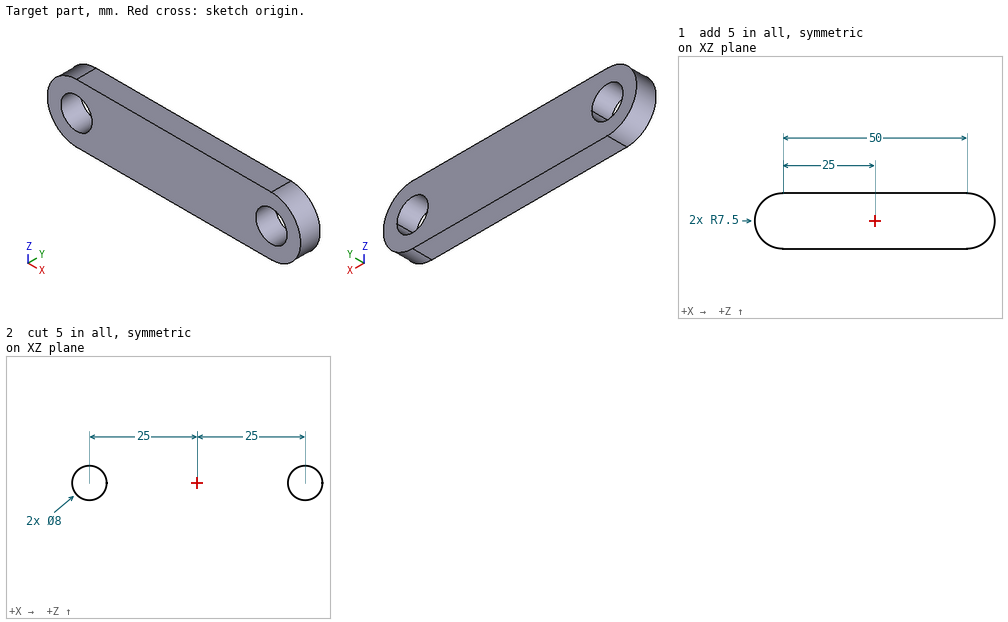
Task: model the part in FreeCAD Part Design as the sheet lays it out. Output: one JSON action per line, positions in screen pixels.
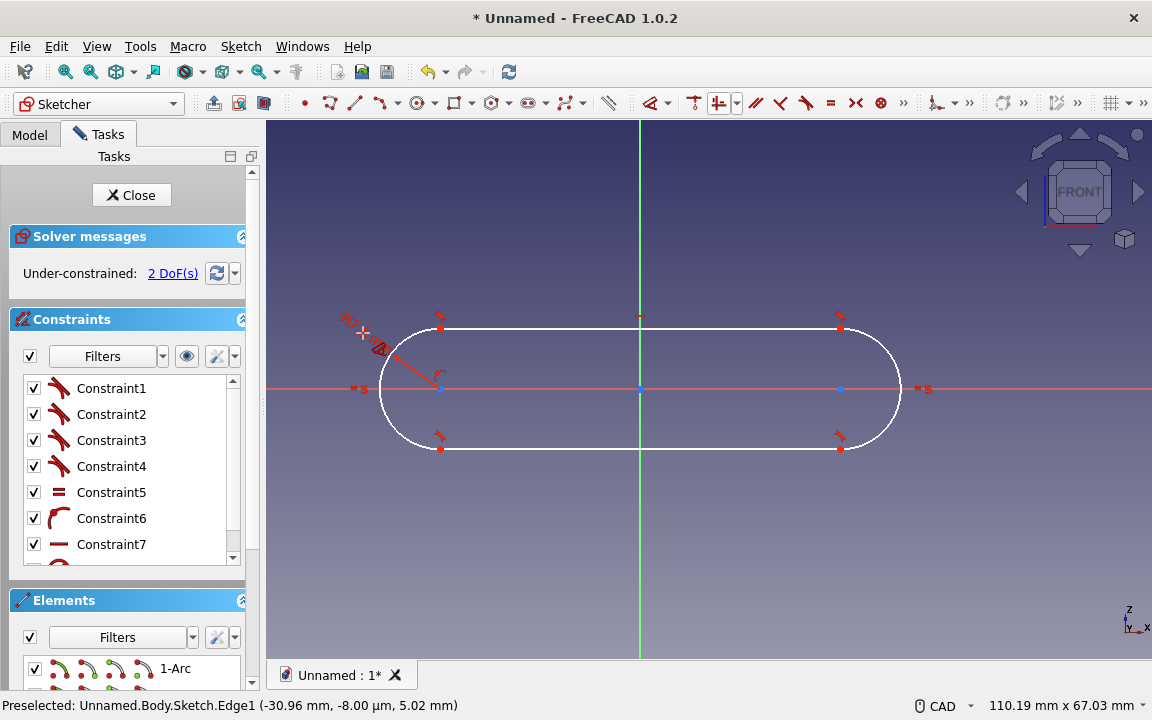
{"action": "left_click", "coordinate": [560, 329]}
{"action": "left_click", "coordinate": [548, 295]}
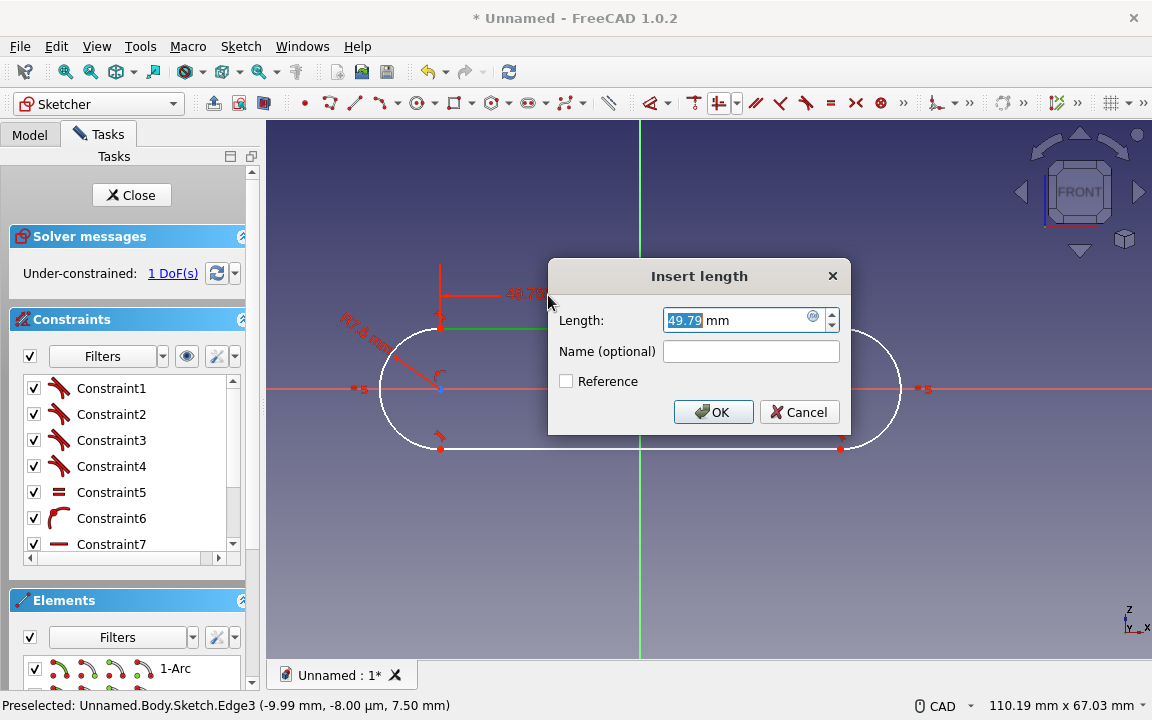
{"action": "type", "text": "50"}
{"action": "key", "text": "Return"}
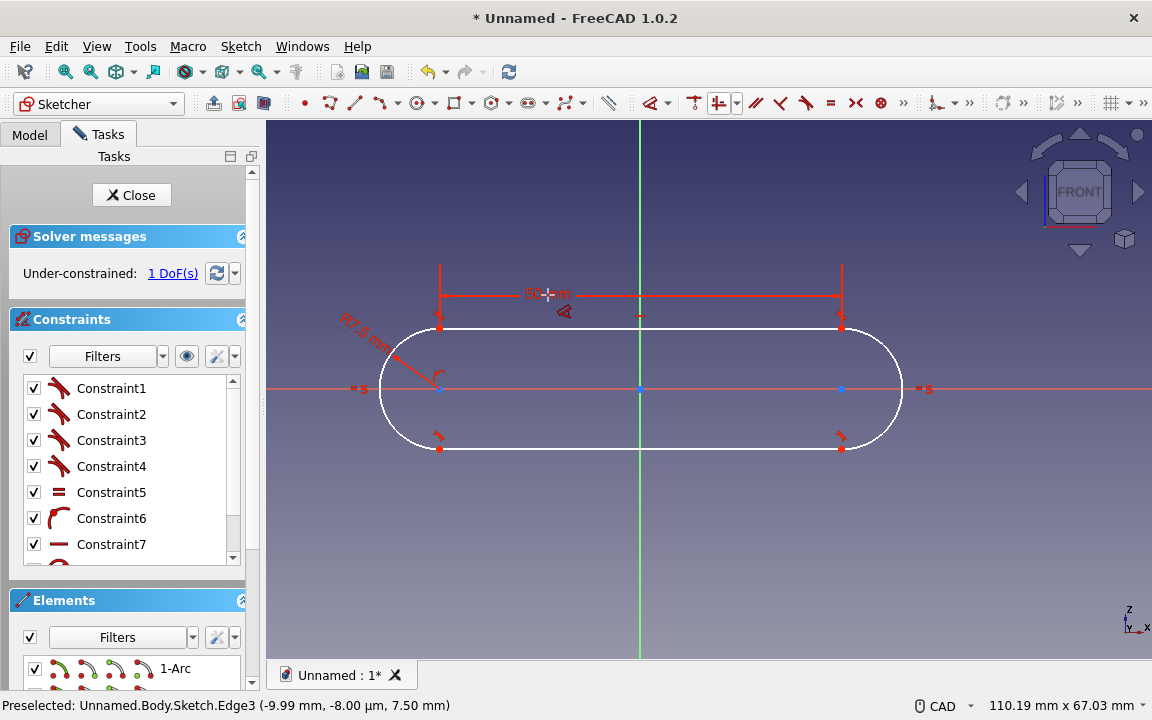
{"action": "left_click", "coordinate": [440, 329]}
{"action": "left_click", "coordinate": [470, 295]}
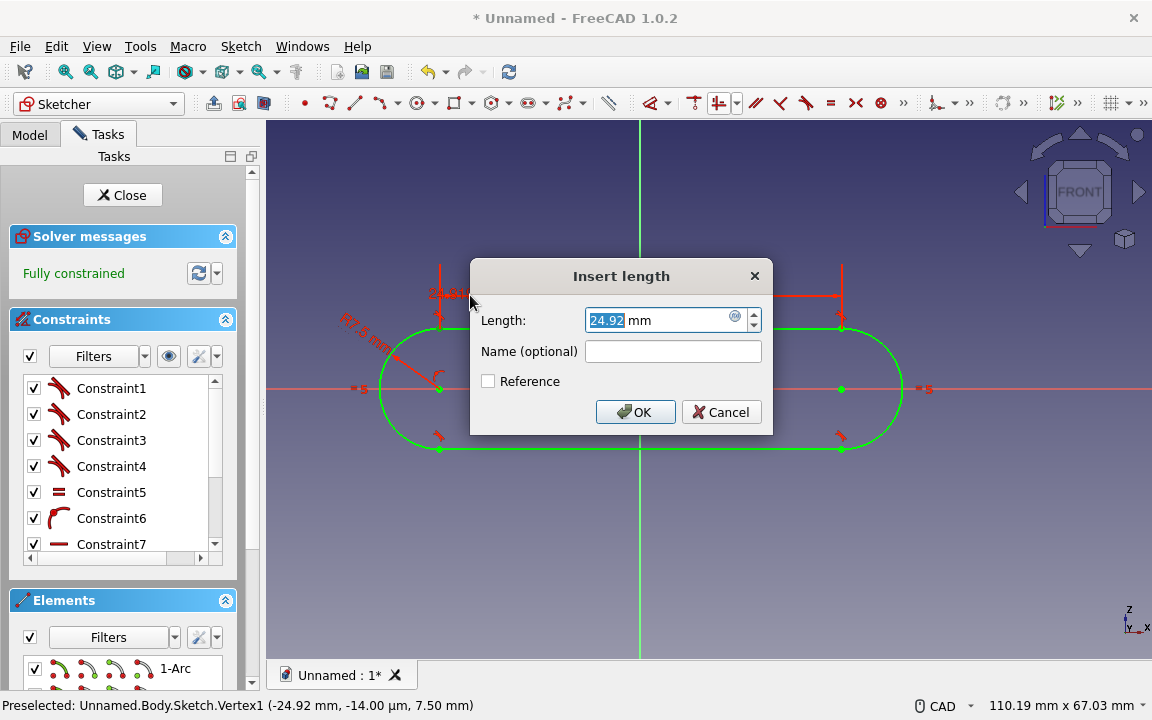
{"action": "type", "text": "25"}
{"action": "key", "text": "Return"}
{"action": "key", "text": "Escape"}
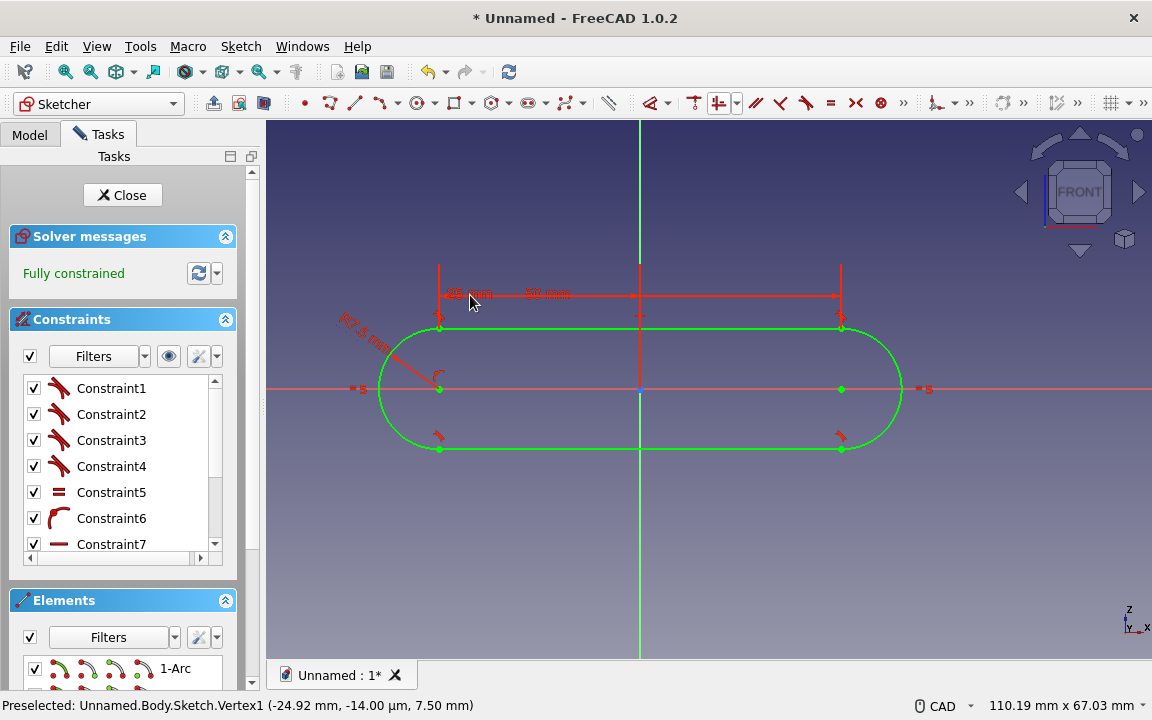
{"action": "left_click", "coordinate": [123, 195]}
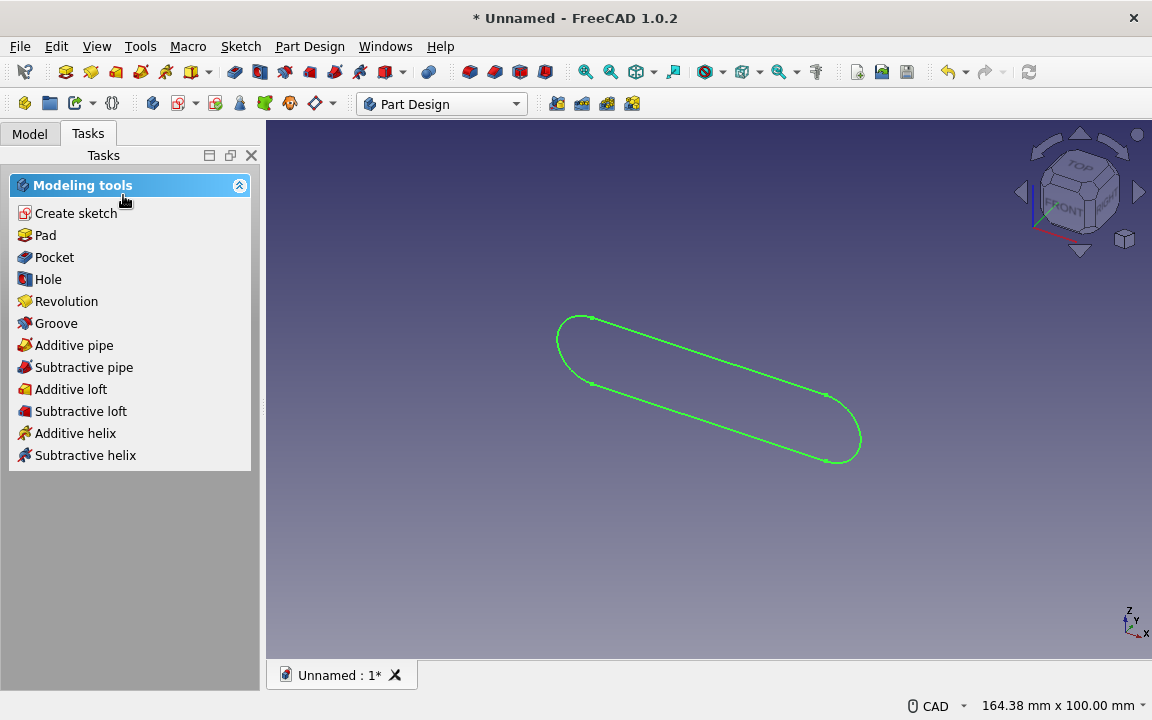
{"action": "left_click", "coordinate": [66, 72]}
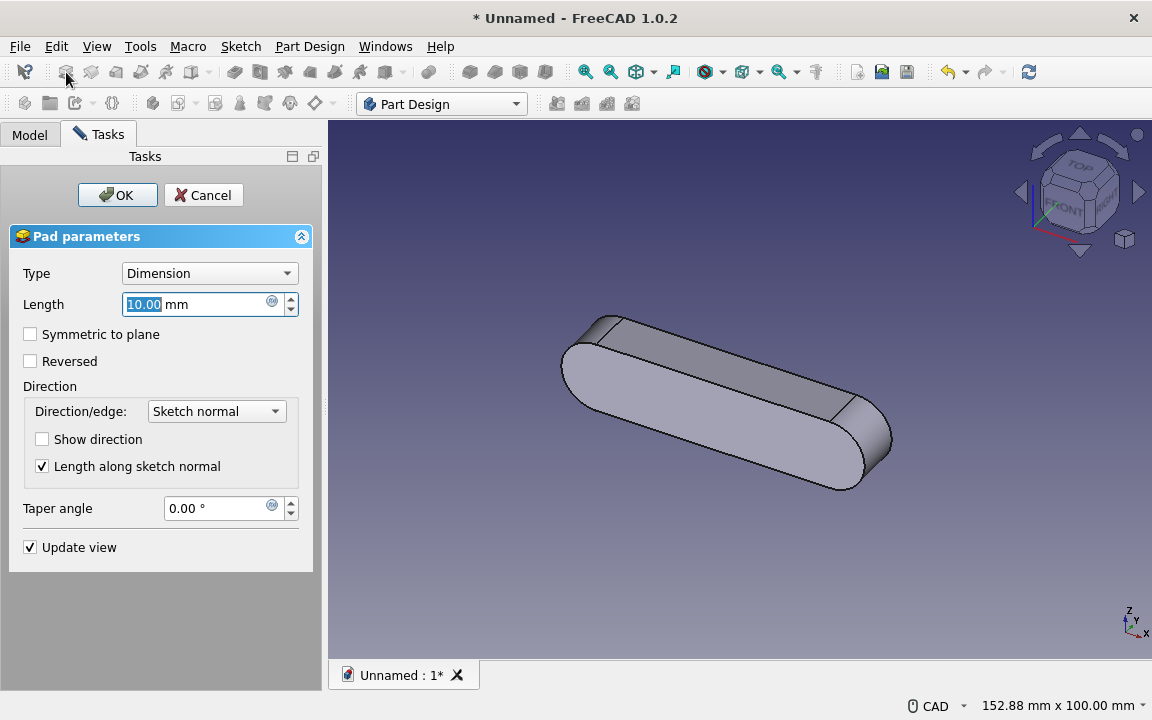
{"action": "type", "text": "5"}
{"action": "key", "text": "Tab"}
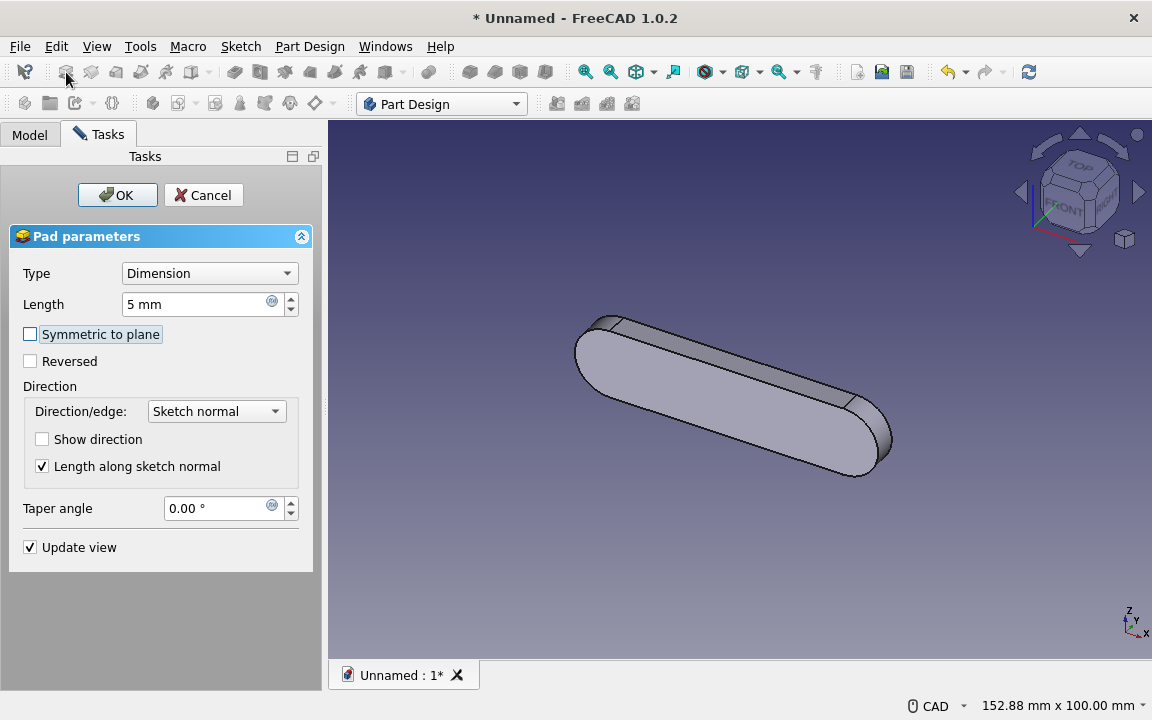
{"action": "left_click", "coordinate": [31, 334]}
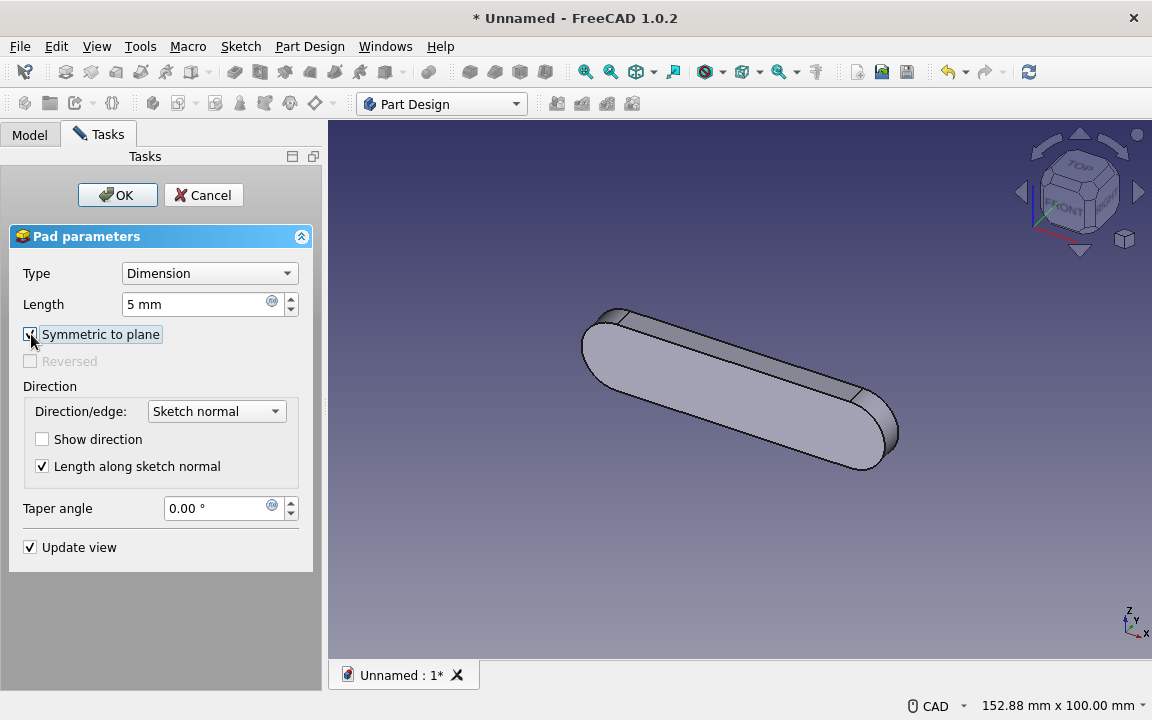
{"action": "left_click", "coordinate": [118, 195]}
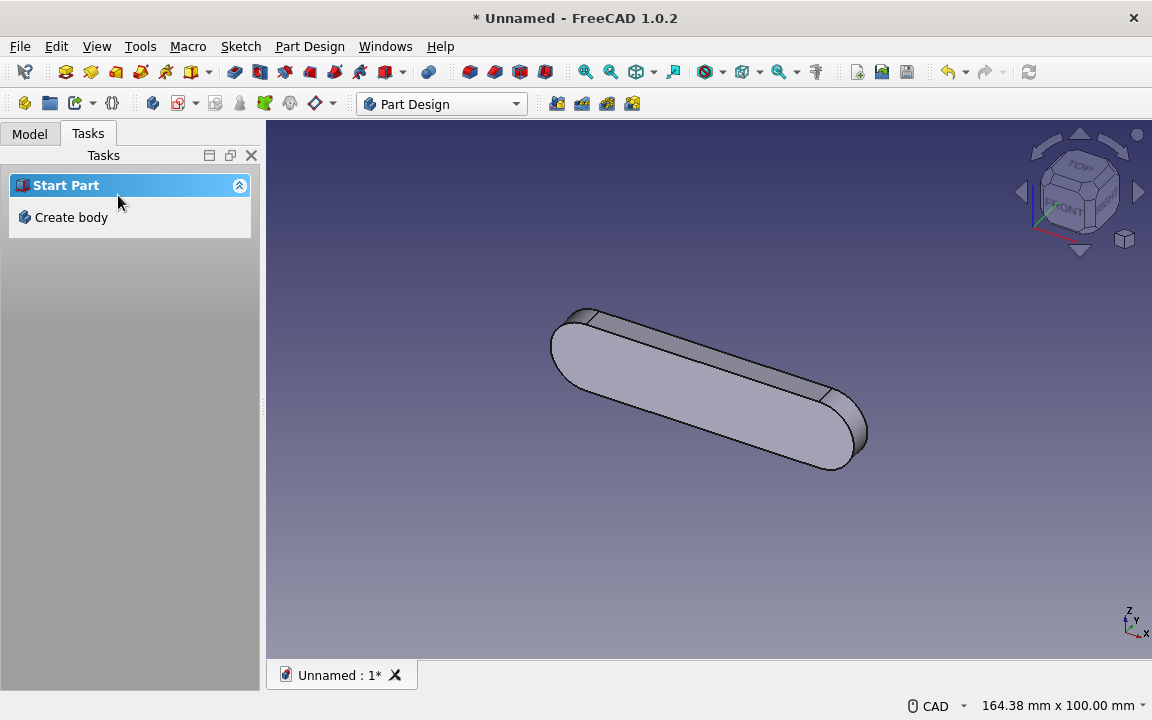
{"action": "left_click", "coordinate": [586, 72]}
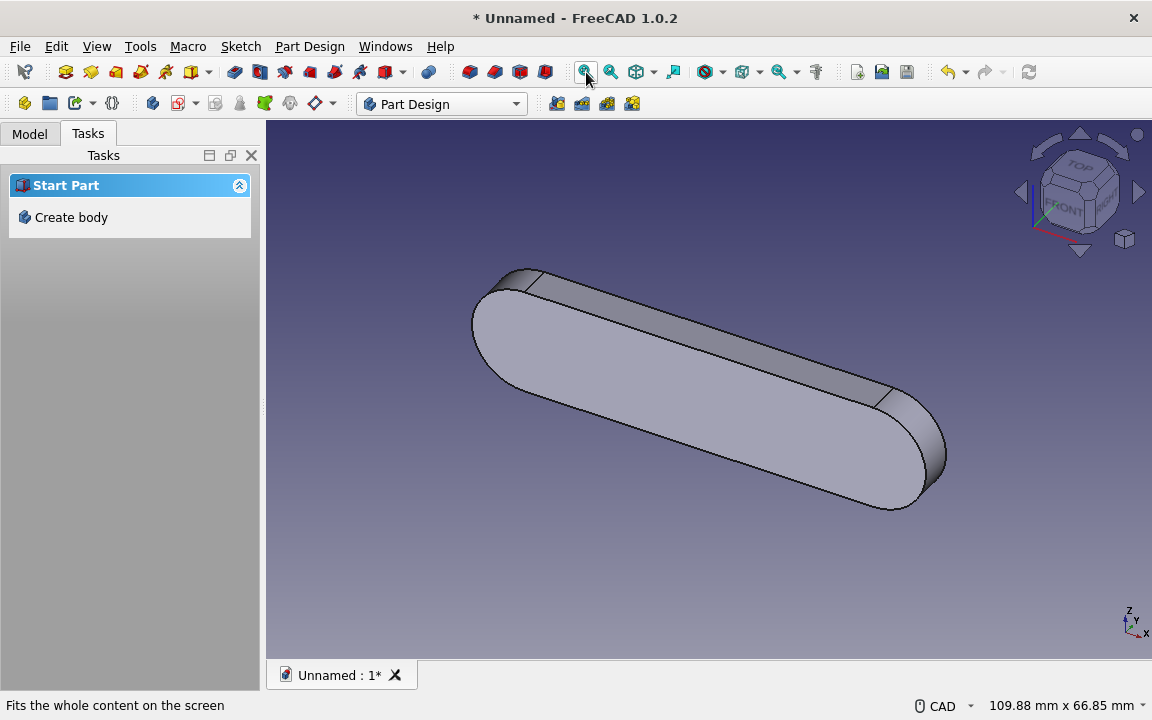
{"action": "left_click", "coordinate": [178, 104]}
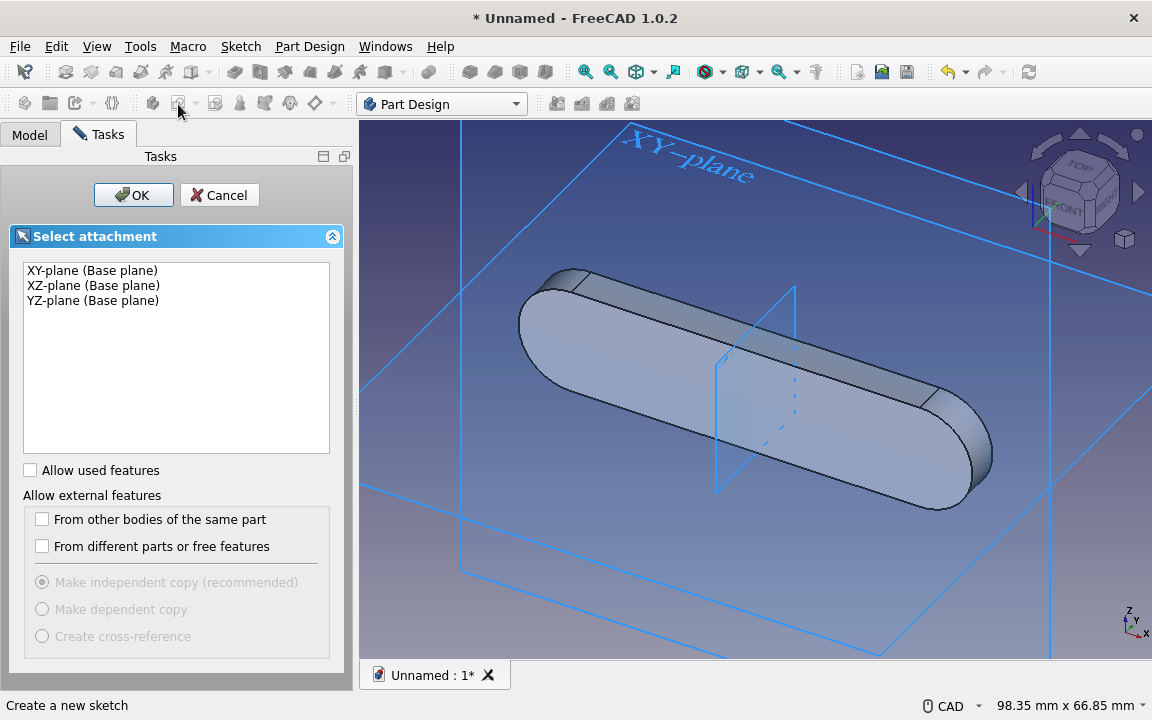
{"action": "left_click", "coordinate": [84, 286]}